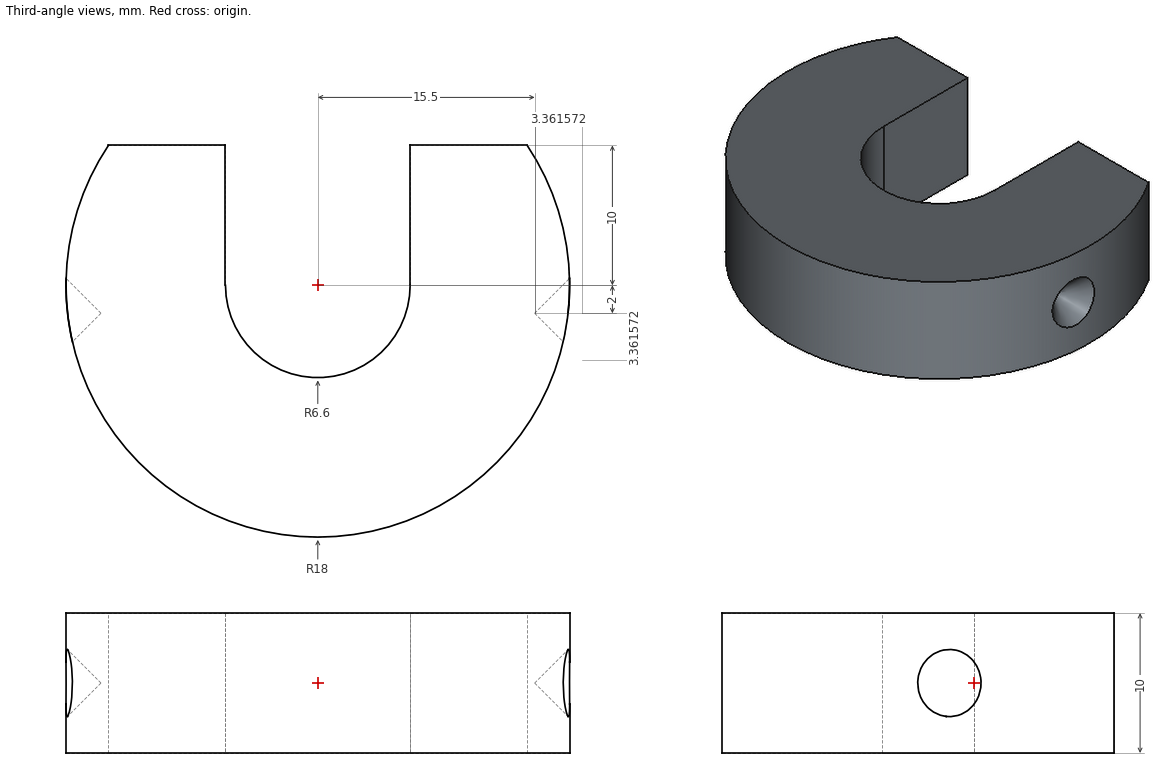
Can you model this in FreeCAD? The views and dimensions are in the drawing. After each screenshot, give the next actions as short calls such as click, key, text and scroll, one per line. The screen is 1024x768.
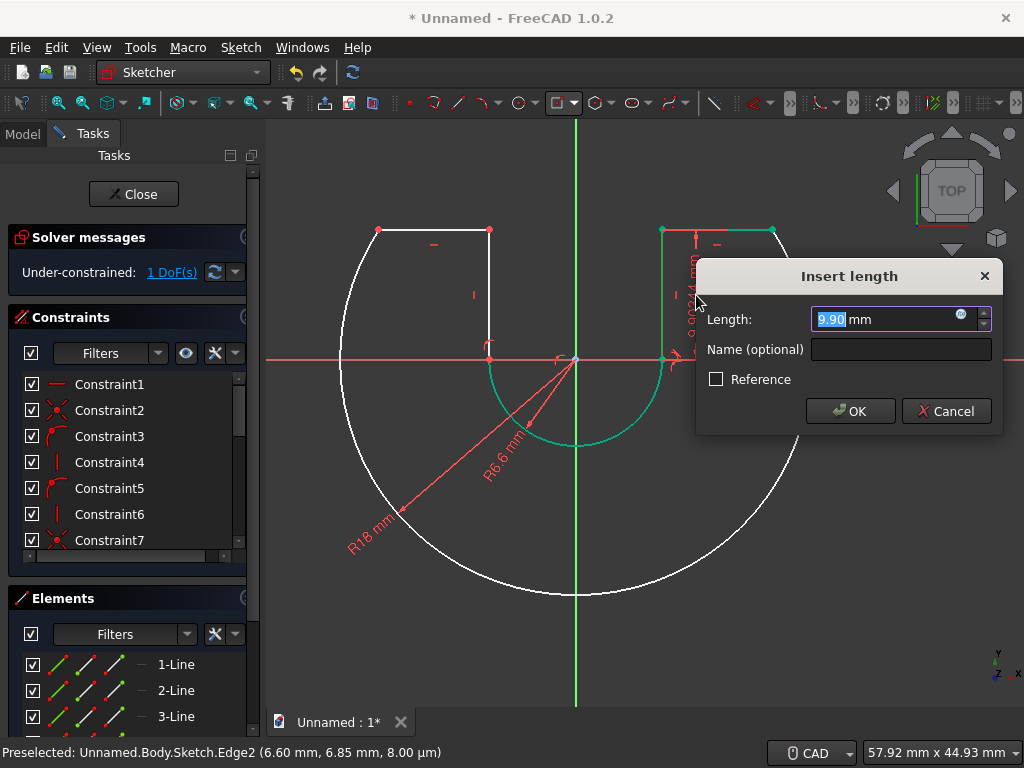
text(10)
key(Return)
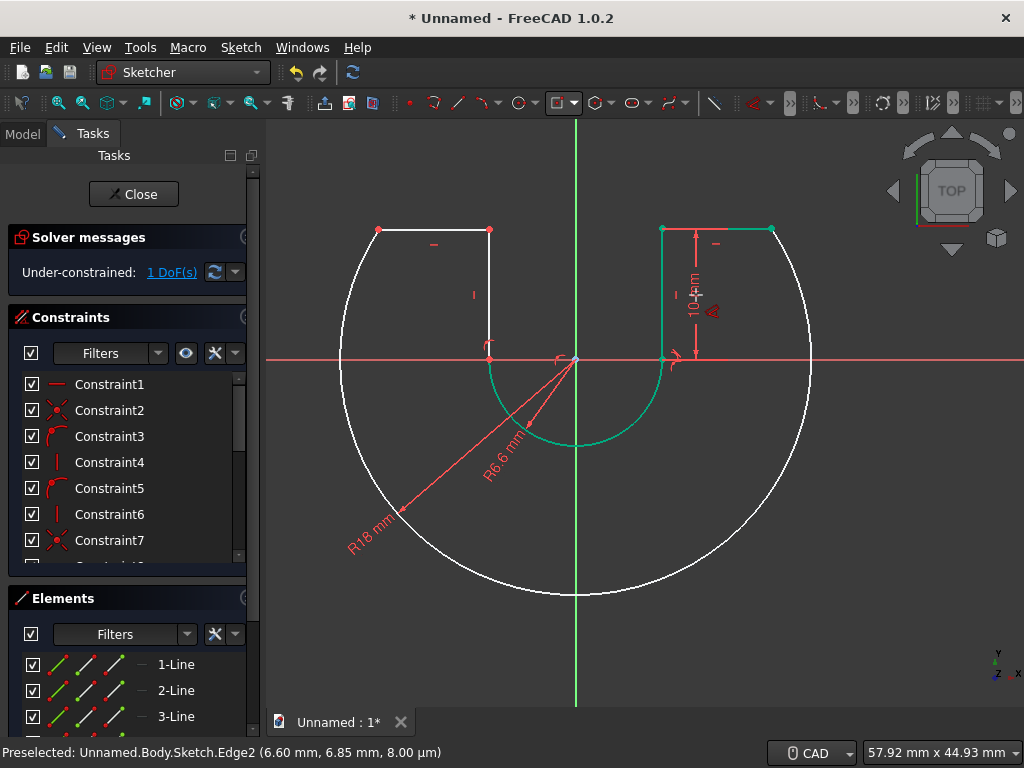
click(489, 321)
click(455, 295)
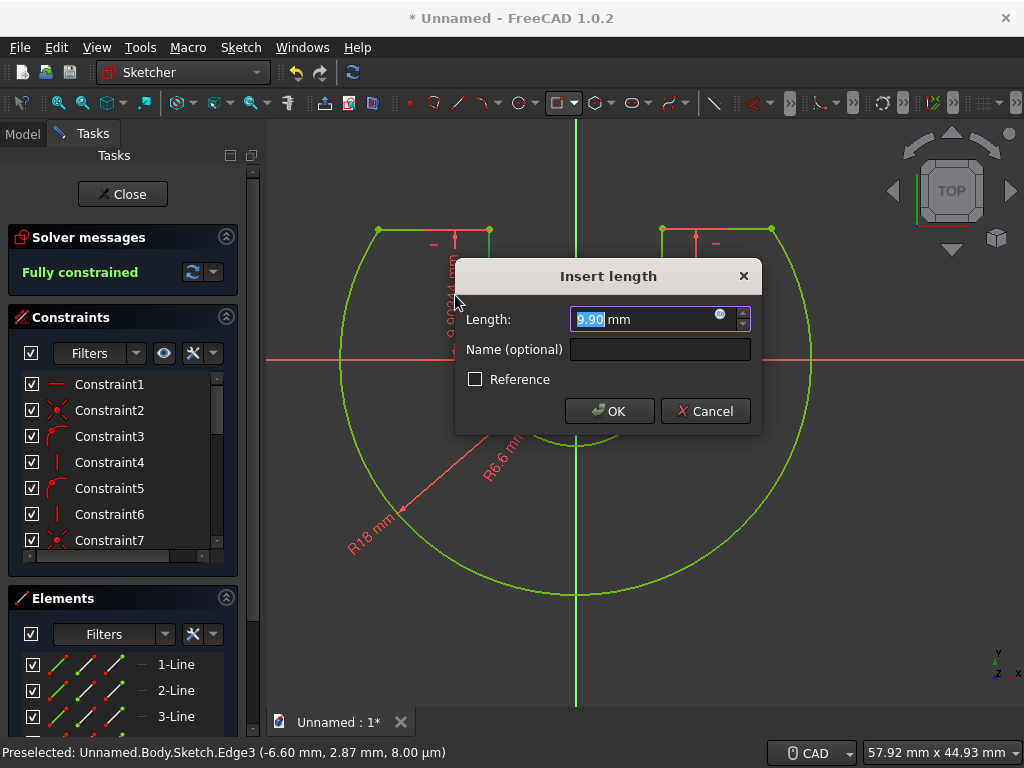
text(10)
key(Return)
key(Escape)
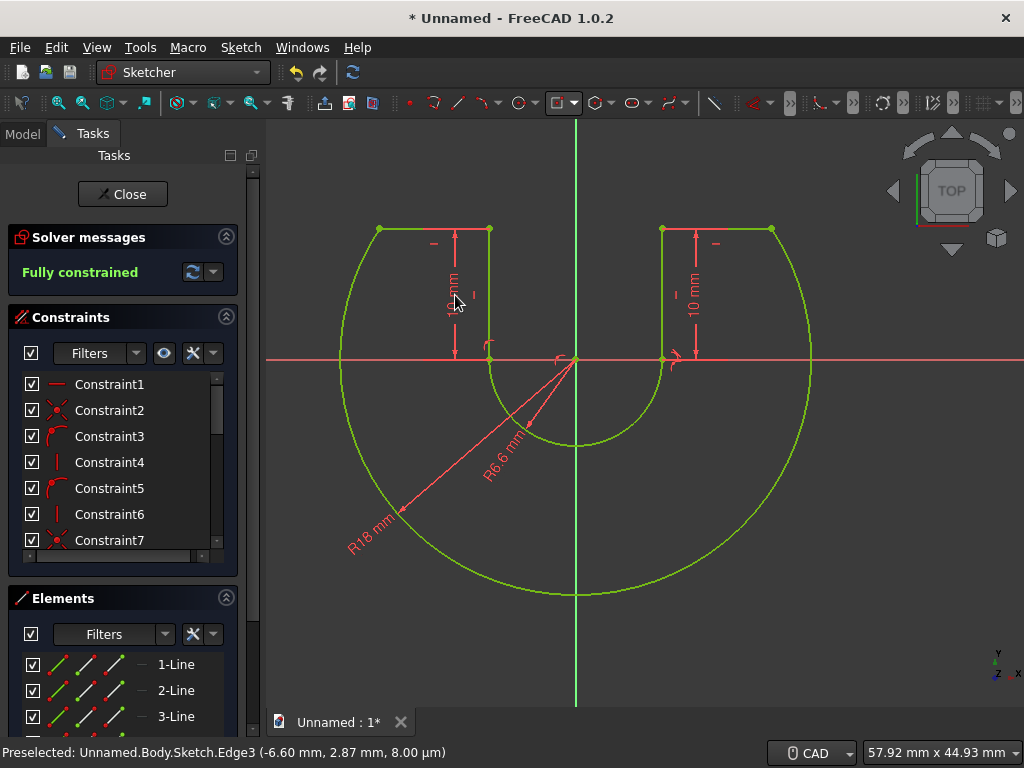
click(123, 194)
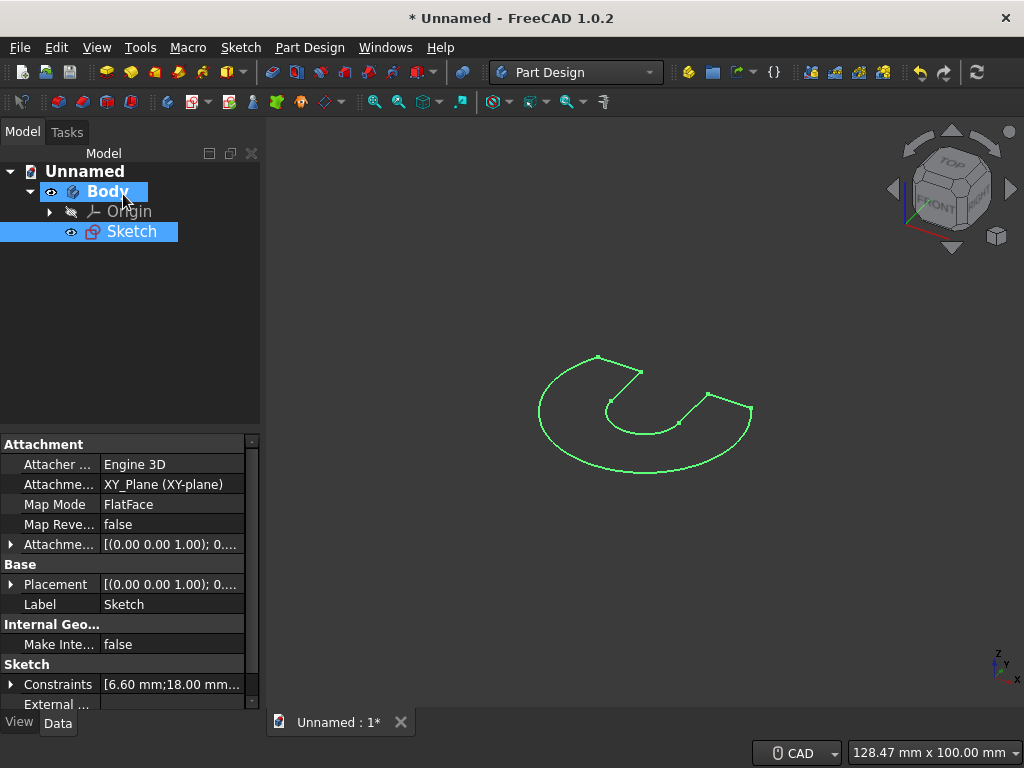
click(108, 72)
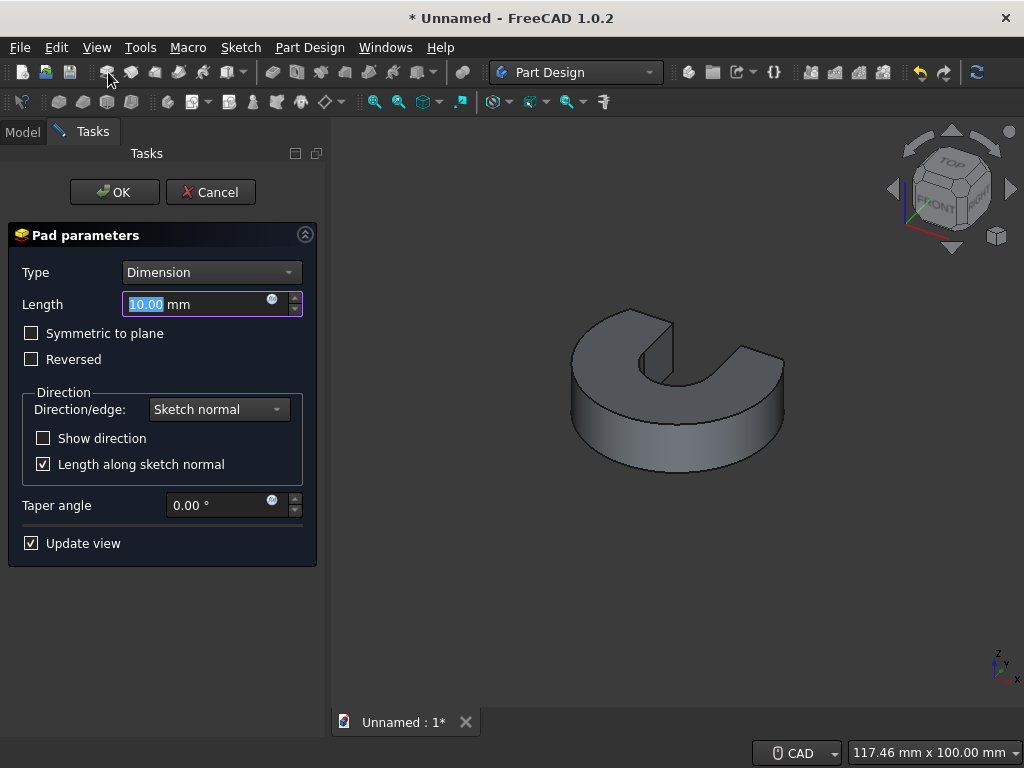
text(10)
key(Tab)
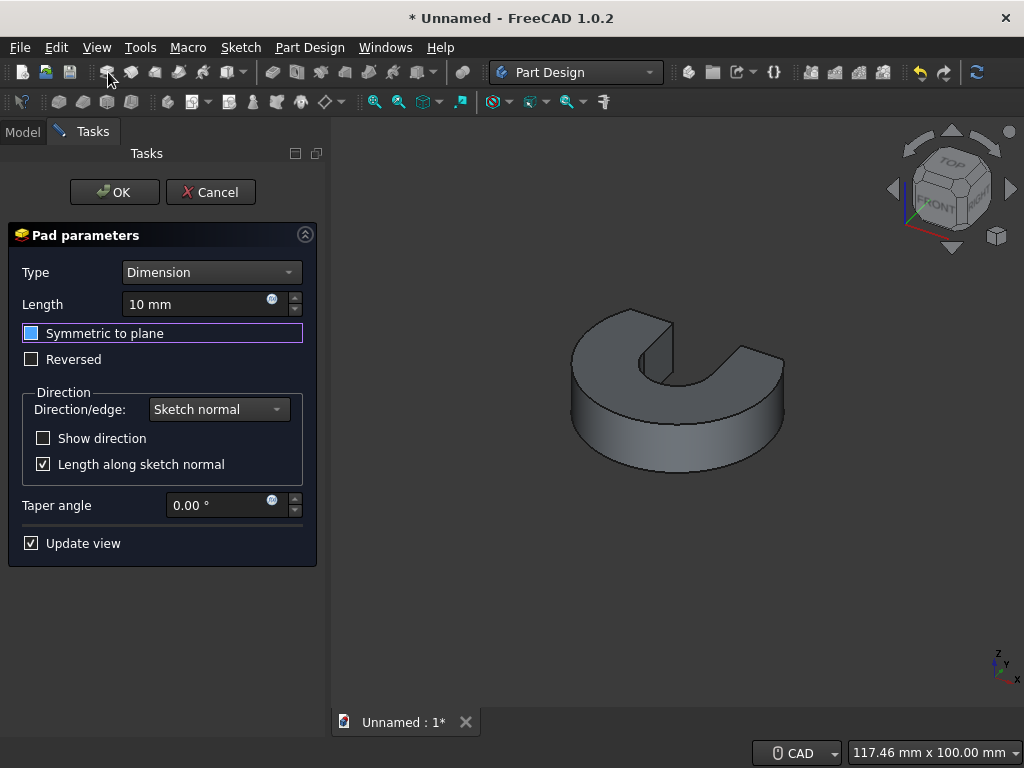
click(30, 333)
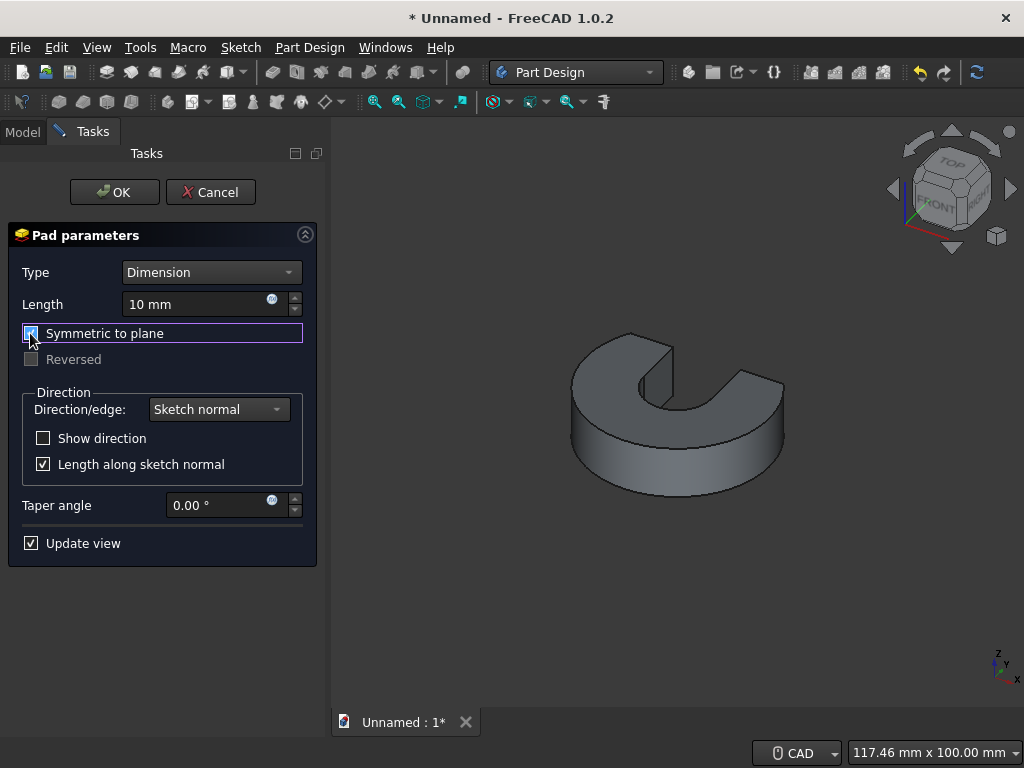
click(115, 192)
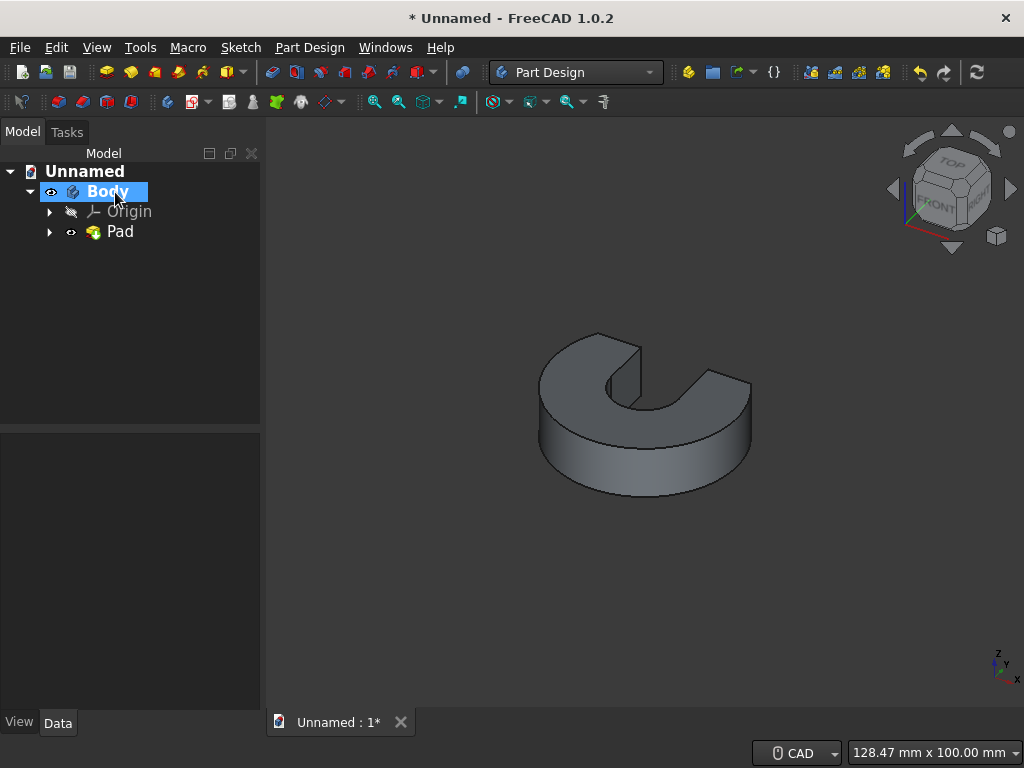
click(376, 102)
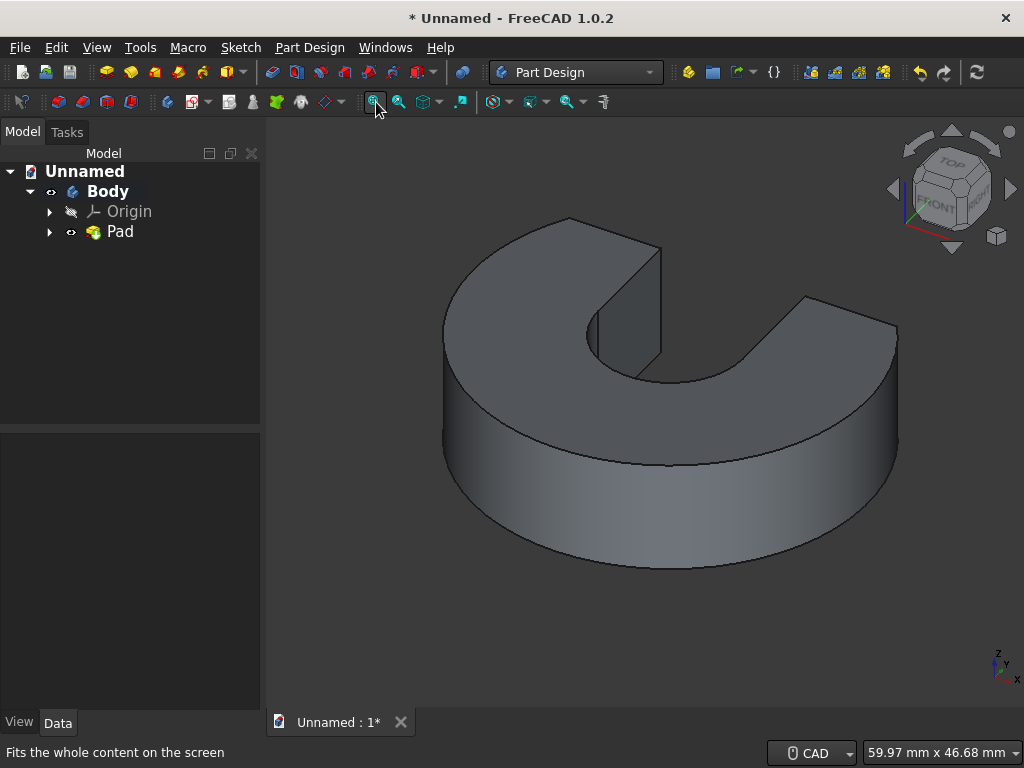
click(192, 102)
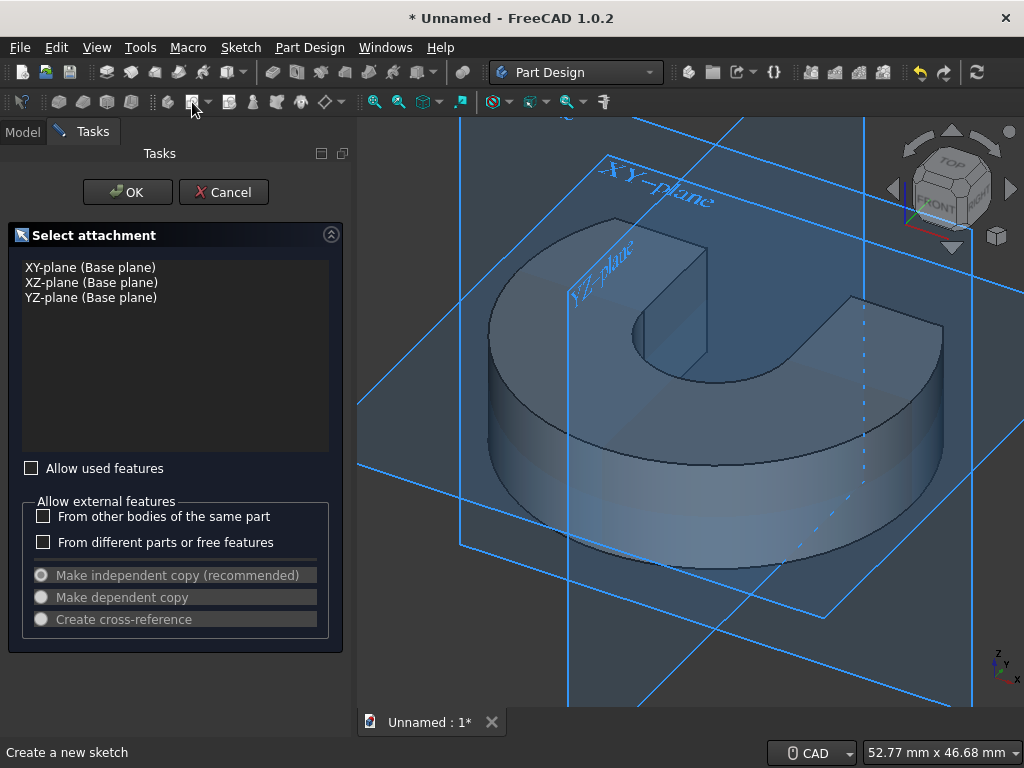
click(82, 268)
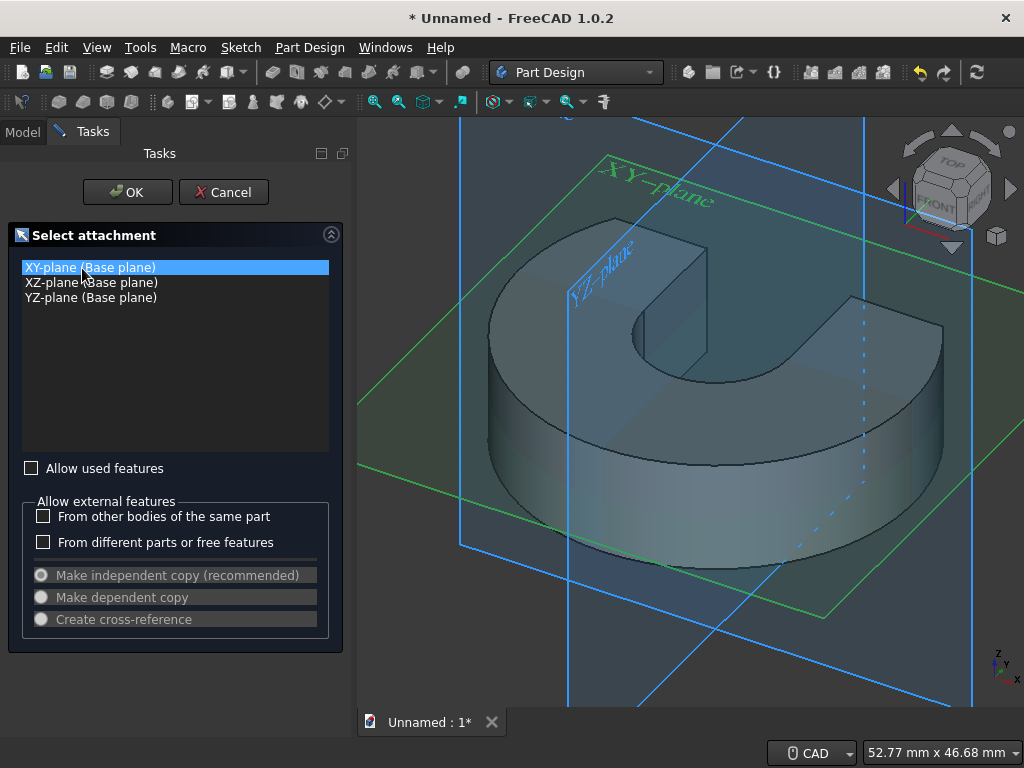
click(128, 192)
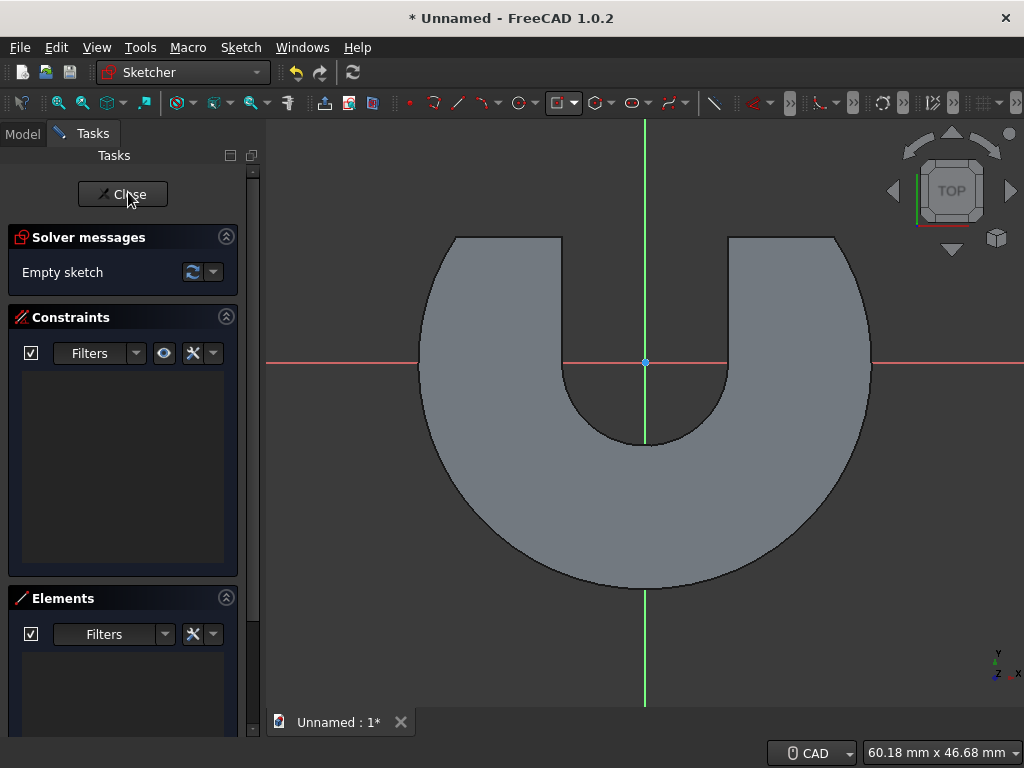
key(q)
key(s)